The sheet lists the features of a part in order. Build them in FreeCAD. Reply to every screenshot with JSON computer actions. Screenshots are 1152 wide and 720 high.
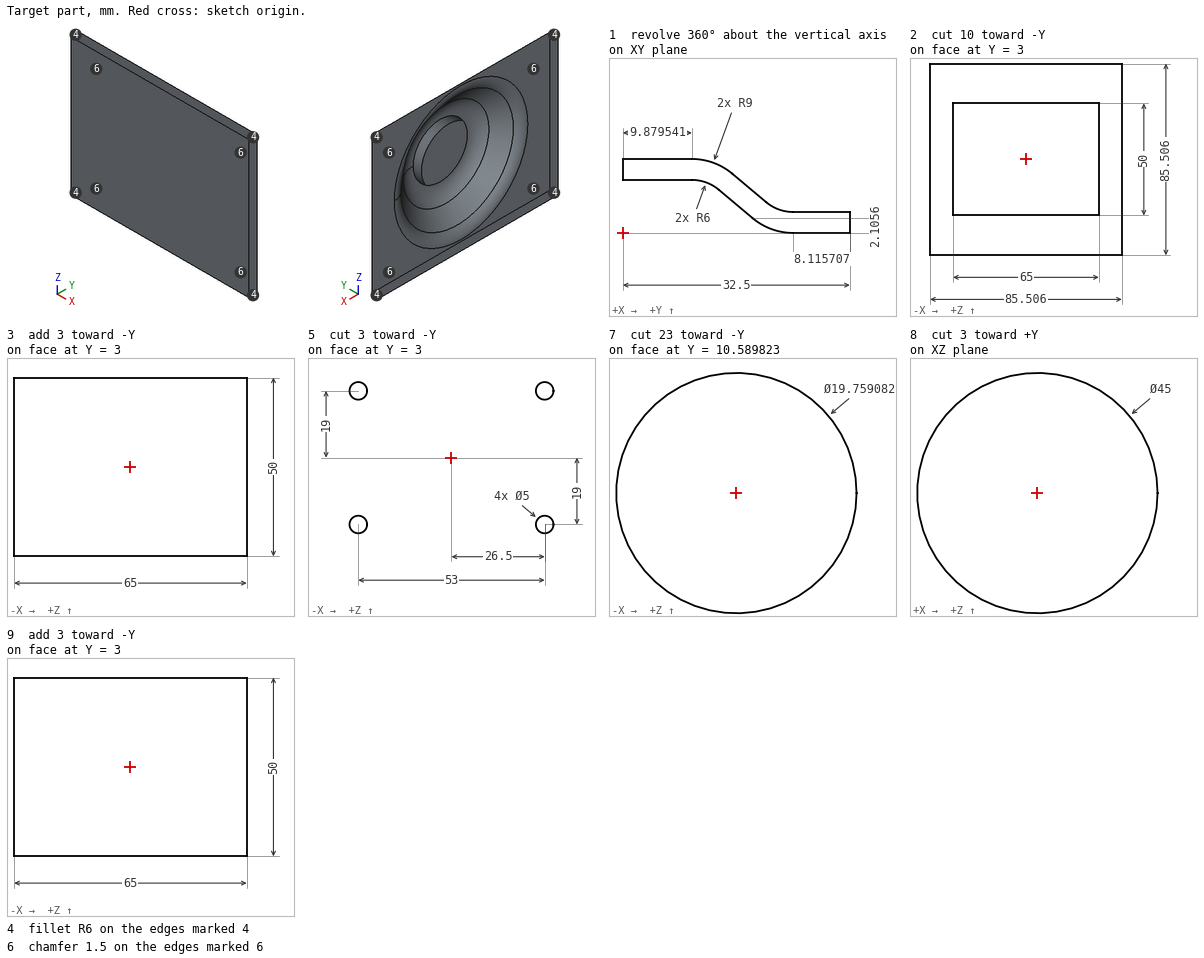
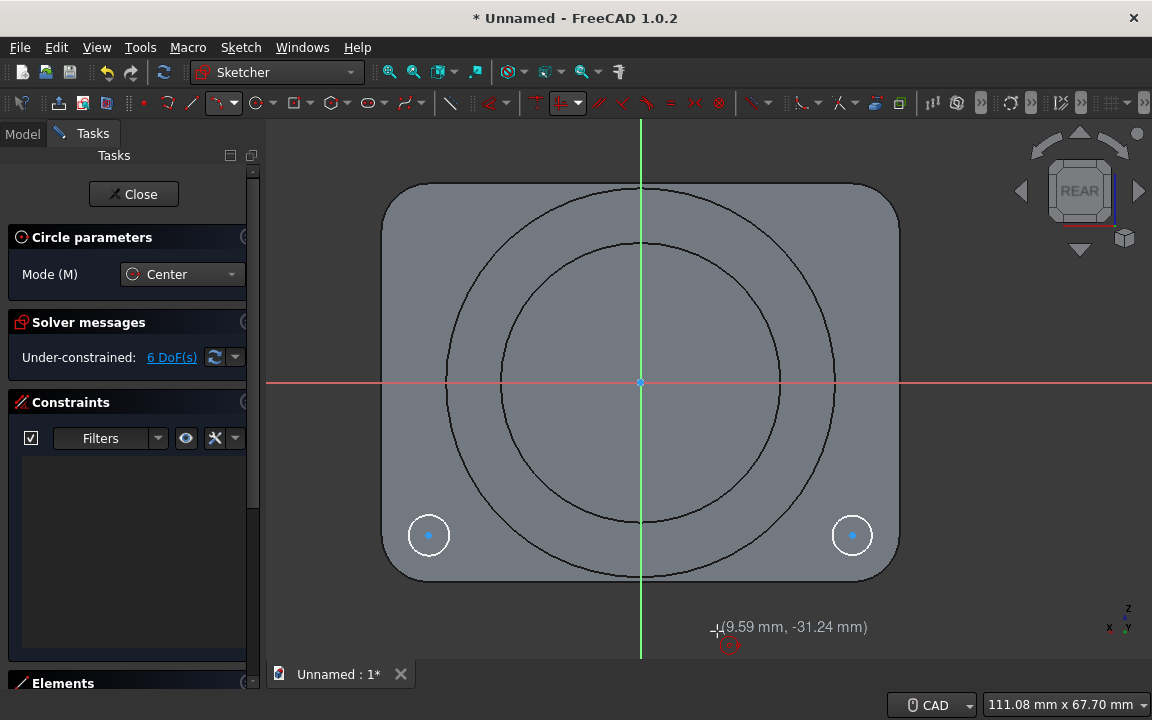
{"action": "left_click", "coordinate": [429, 231]}
{"action": "left_click", "coordinate": [443, 217]}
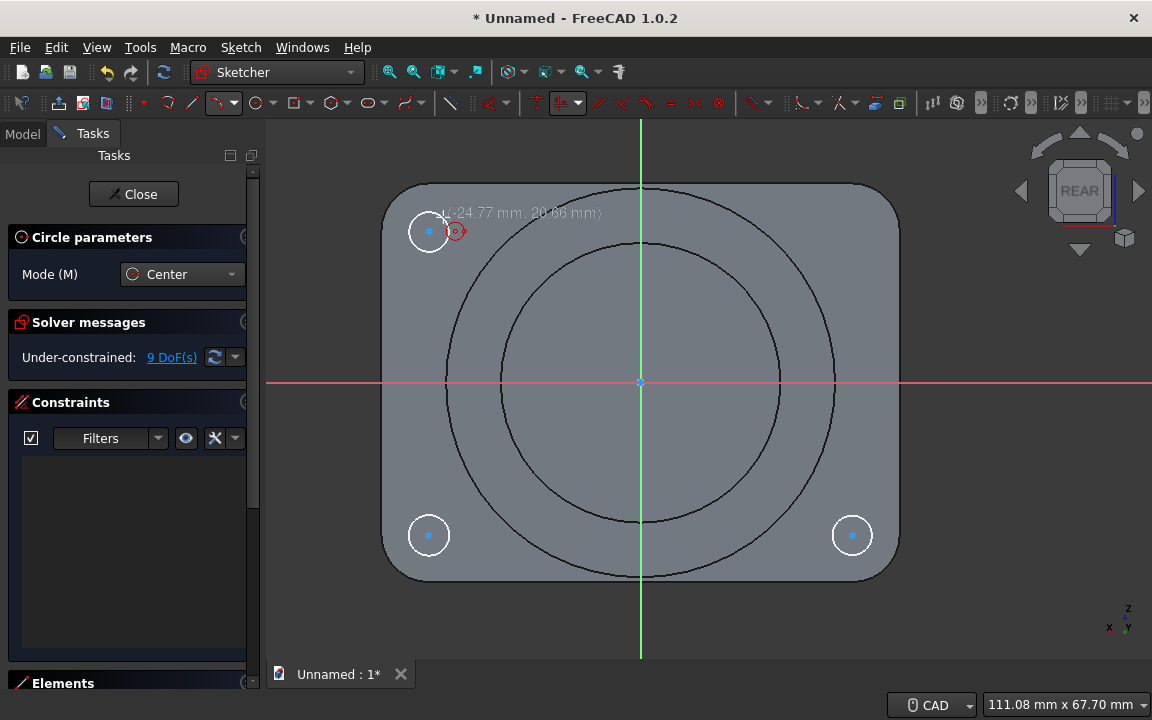
{"action": "left_click", "coordinate": [852, 231]}
{"action": "left_click", "coordinate": [866, 217]}
{"action": "key", "text": "Escape"}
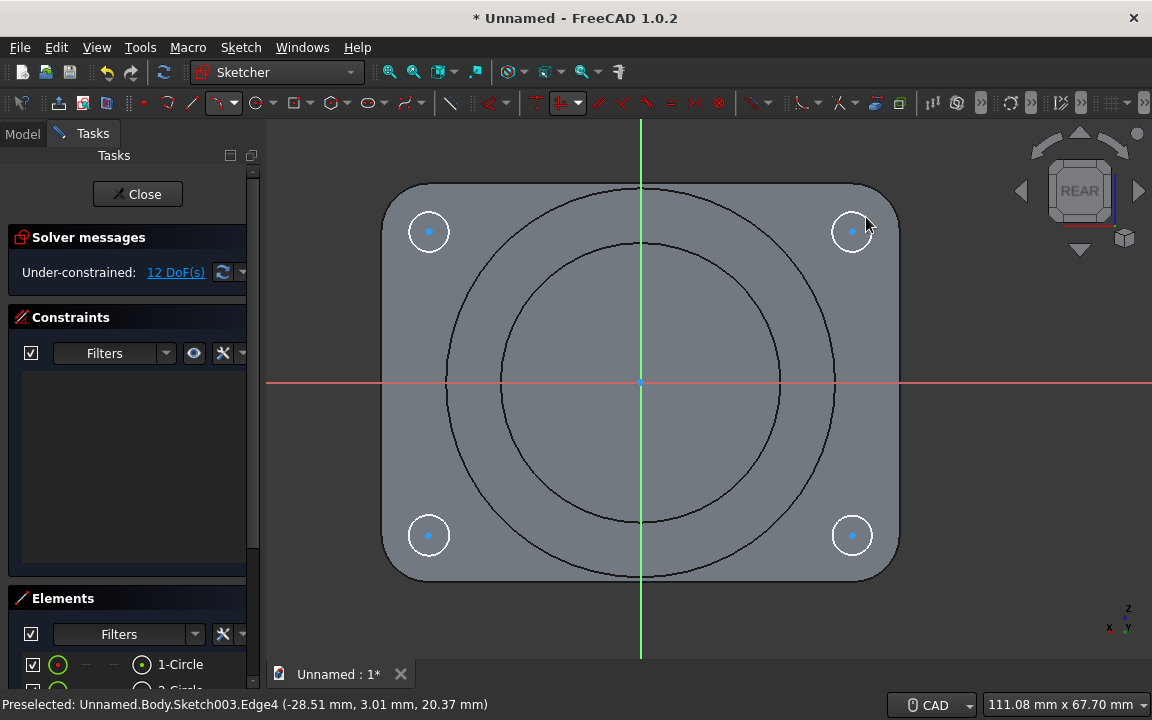
{"action": "left_click", "coordinate": [866, 521]}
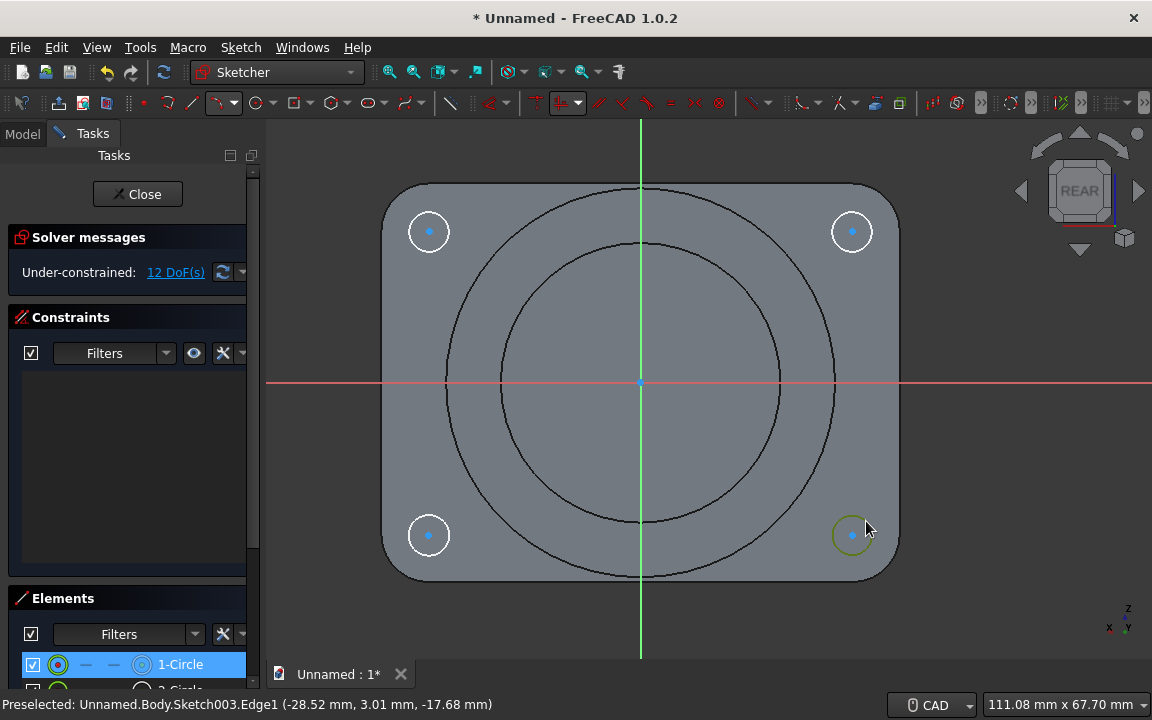
{"action": "left_click", "coordinate": [443, 521]}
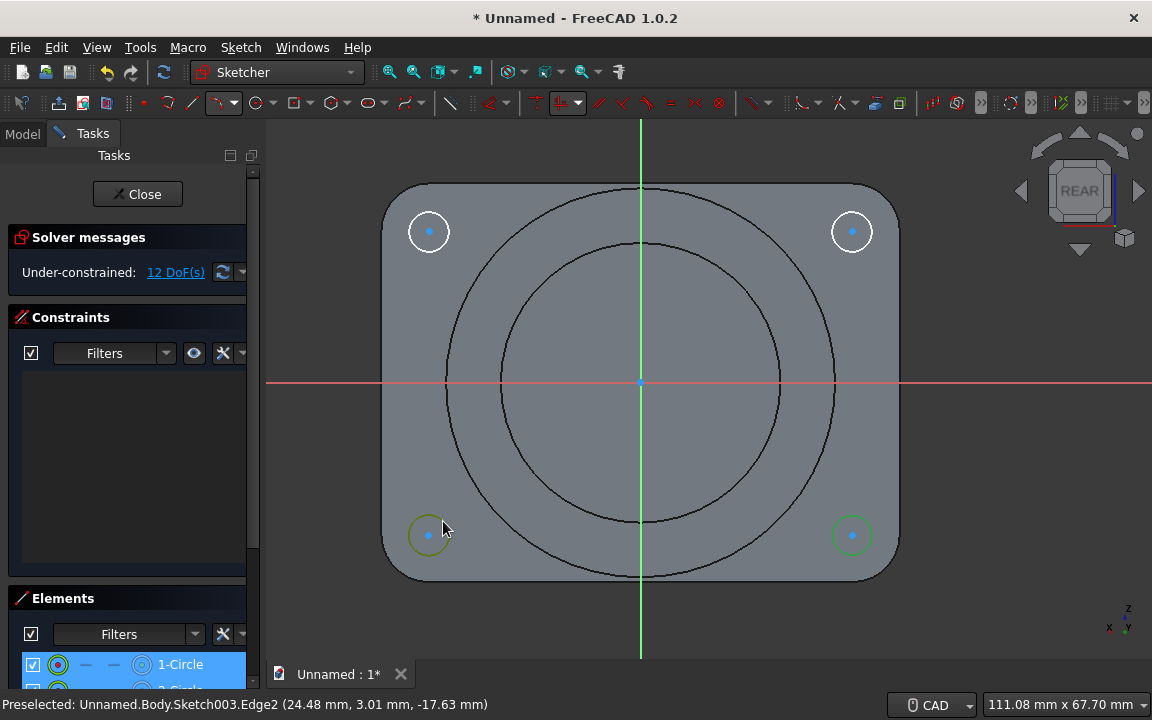
{"action": "left_click", "coordinate": [443, 218]}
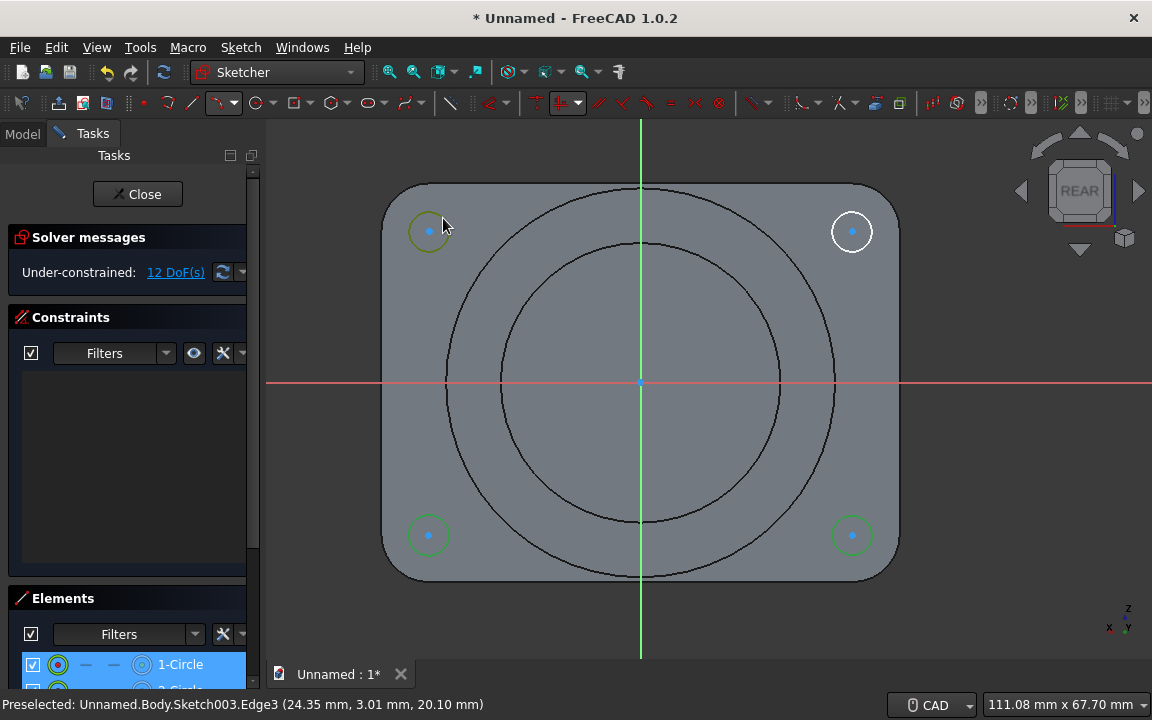
{"action": "left_click", "coordinate": [866, 218]}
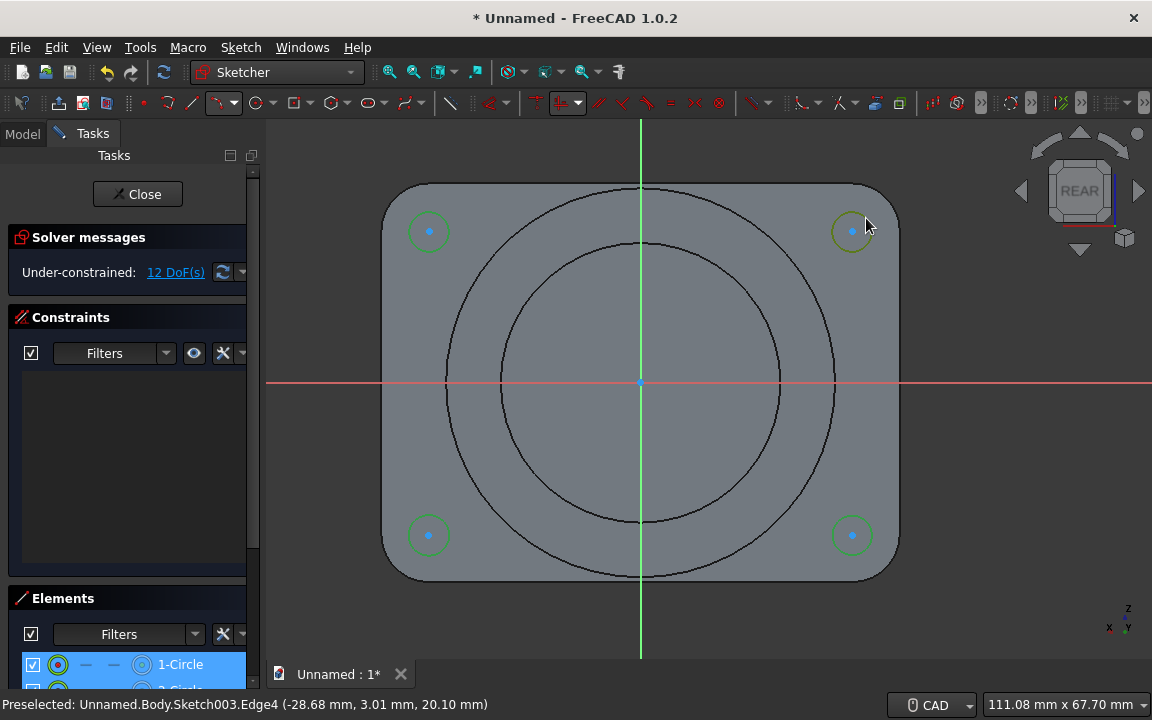
{"action": "left_click", "coordinate": [672, 104]}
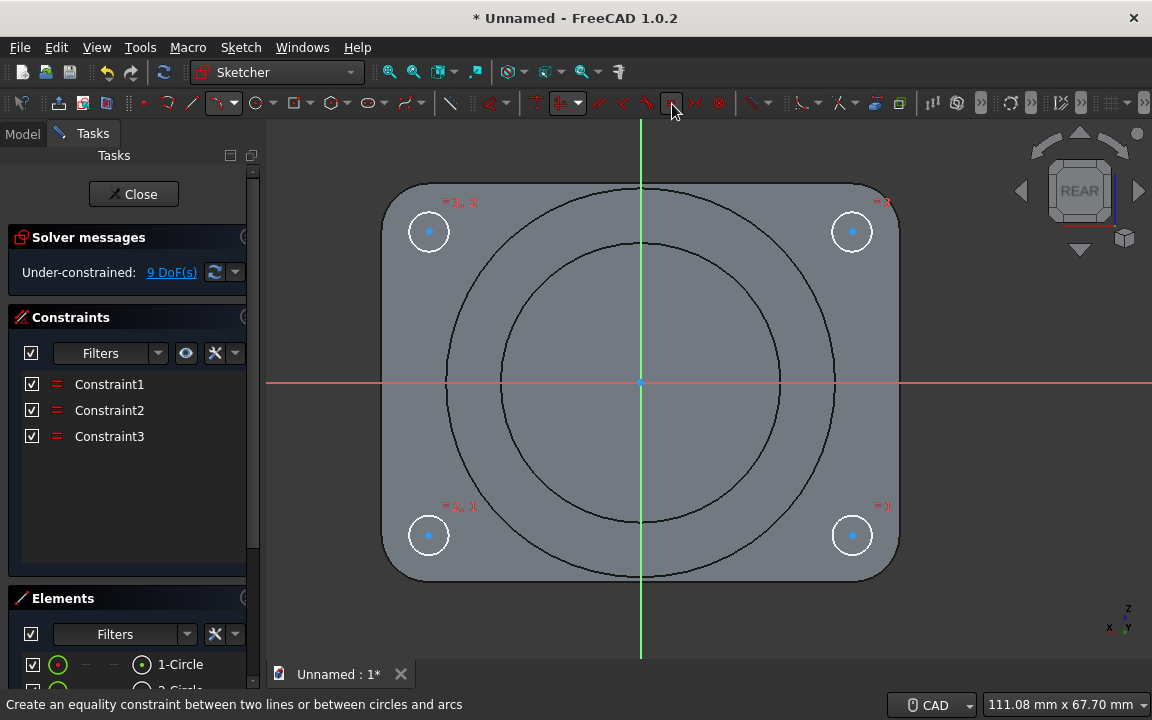
{"action": "left_click", "coordinate": [852, 535]}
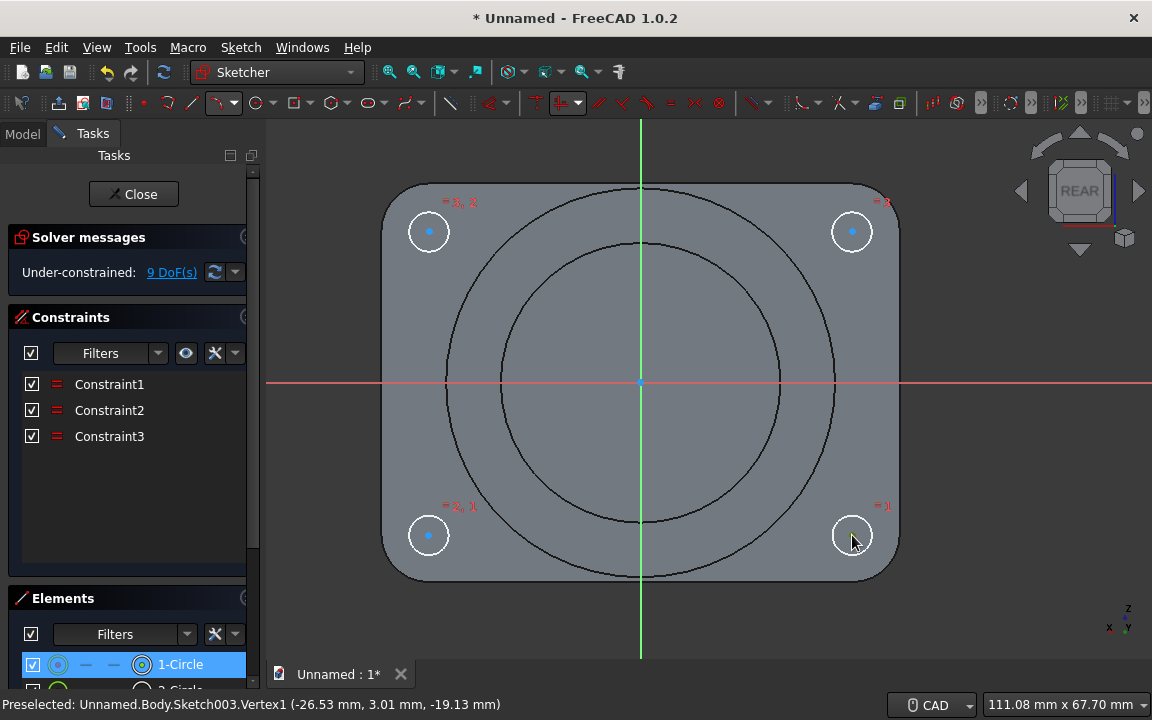
{"action": "left_click", "coordinate": [429, 535]}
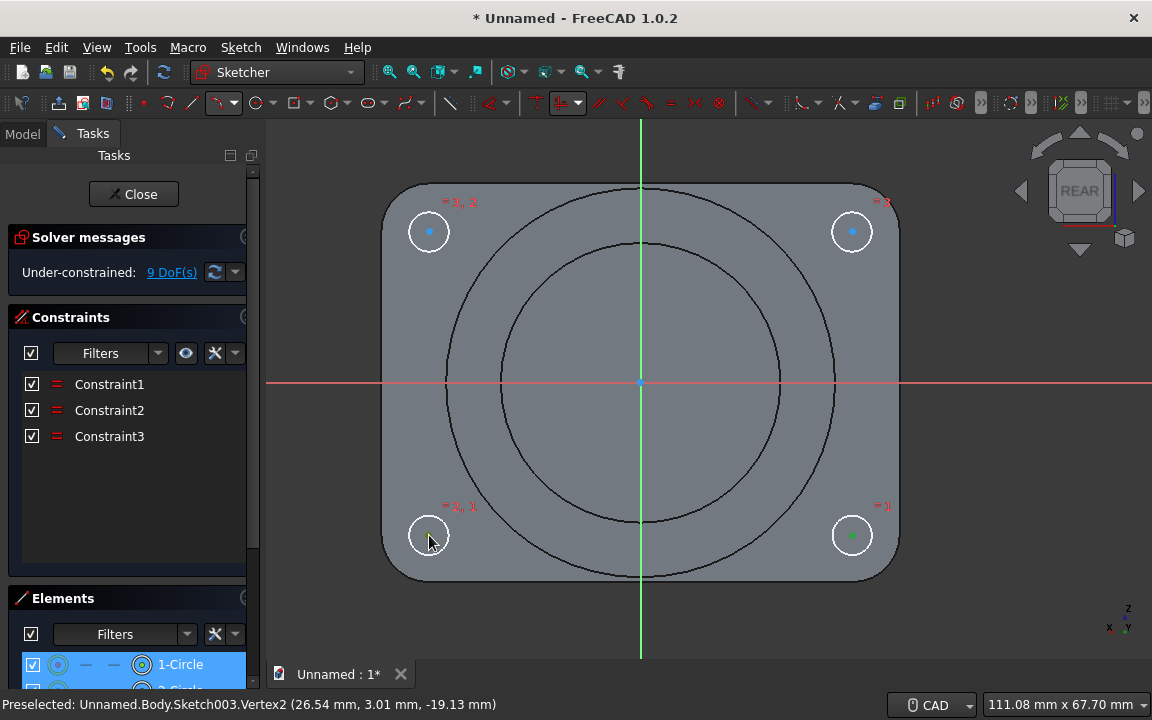
{"action": "left_click", "coordinate": [580, 104]}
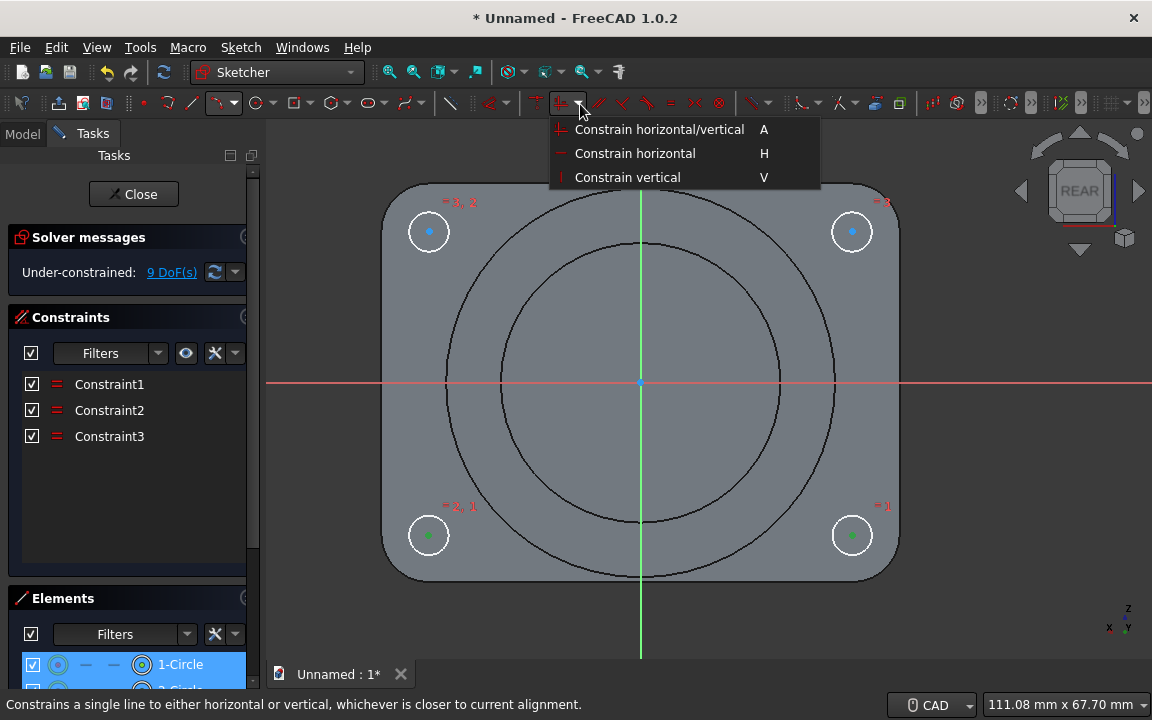
{"action": "left_click", "coordinate": [685, 153]}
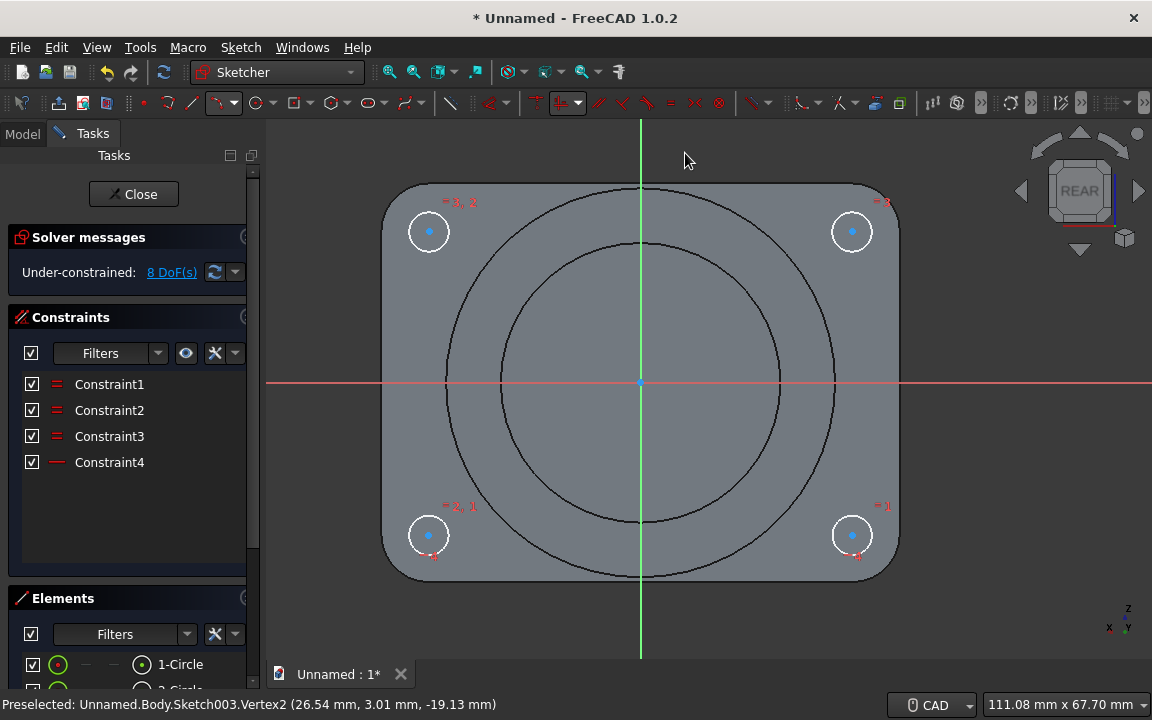
{"action": "left_click", "coordinate": [429, 535]}